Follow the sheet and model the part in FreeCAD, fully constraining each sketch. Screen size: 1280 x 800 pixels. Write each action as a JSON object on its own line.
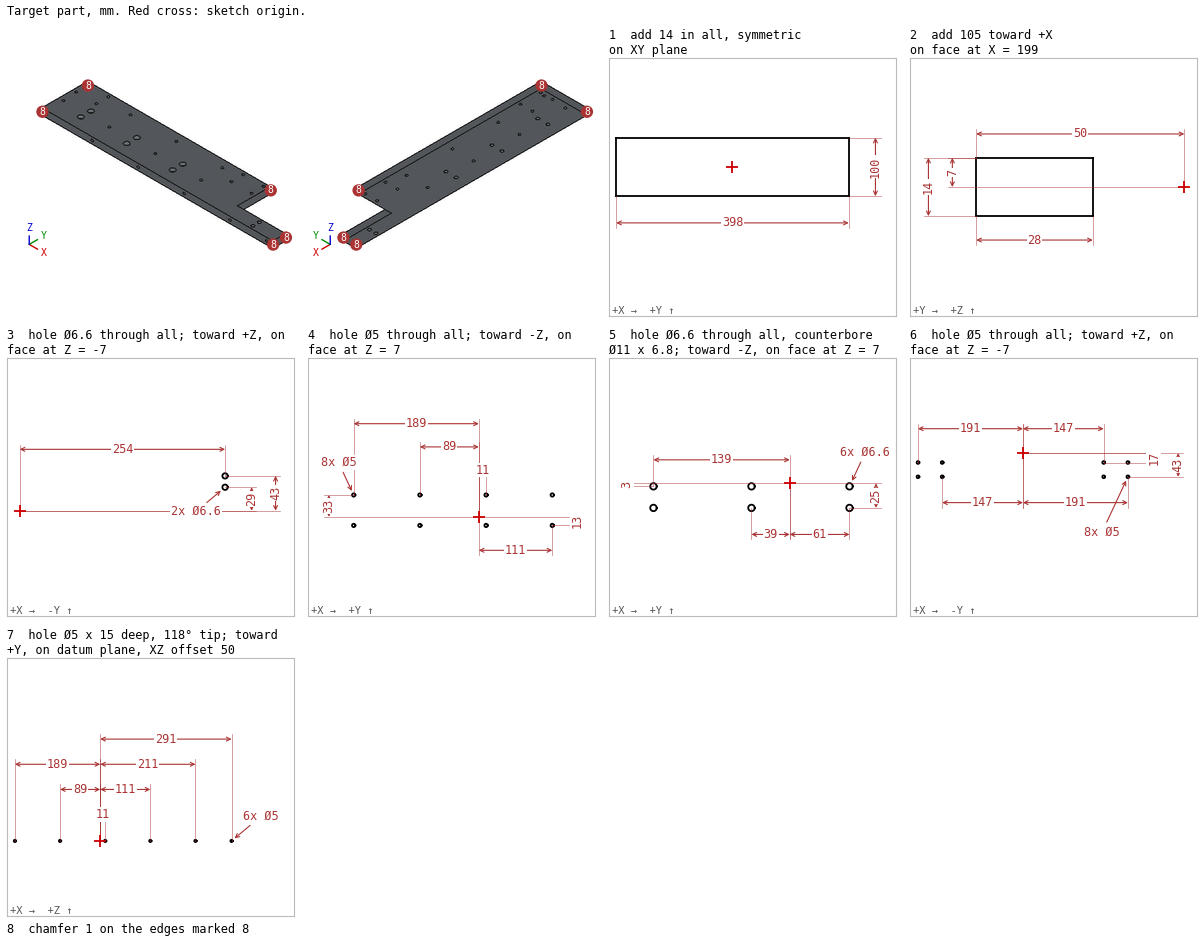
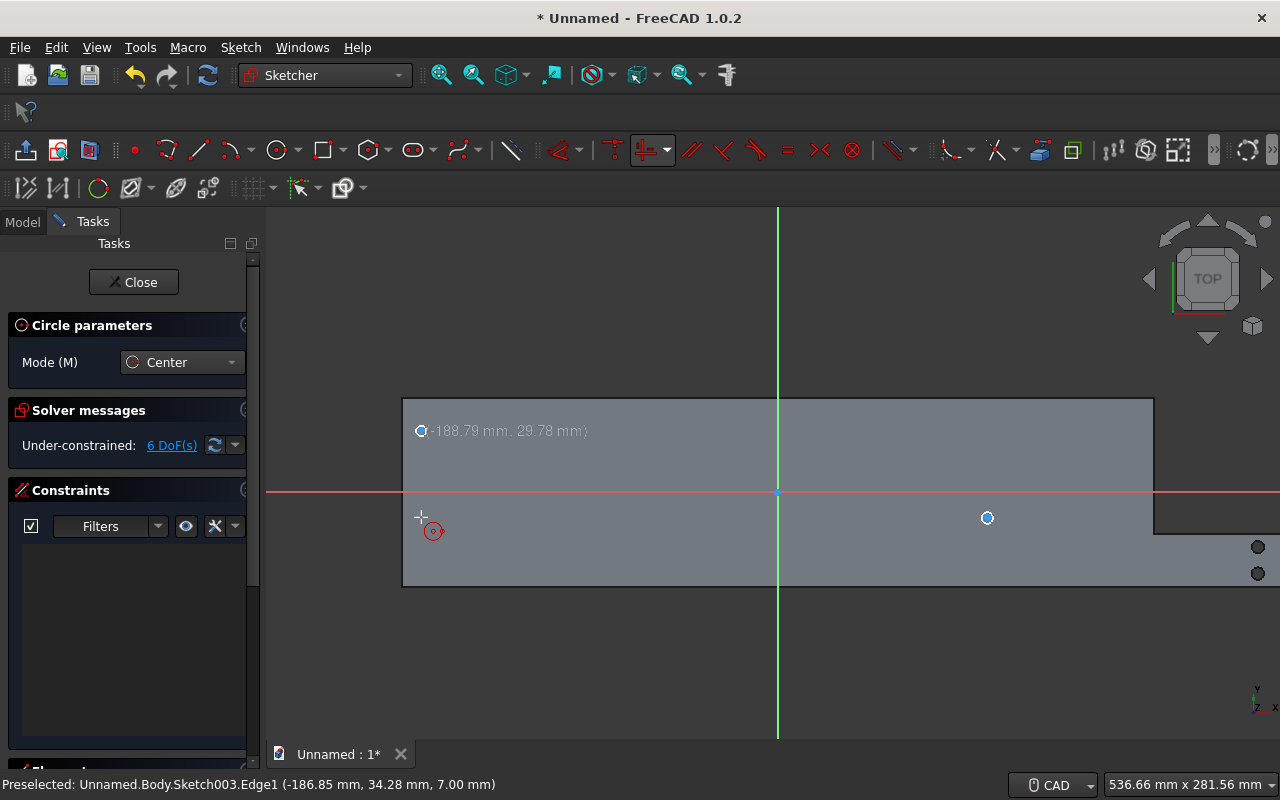
{"action": "left_click", "coordinate": [421, 517]}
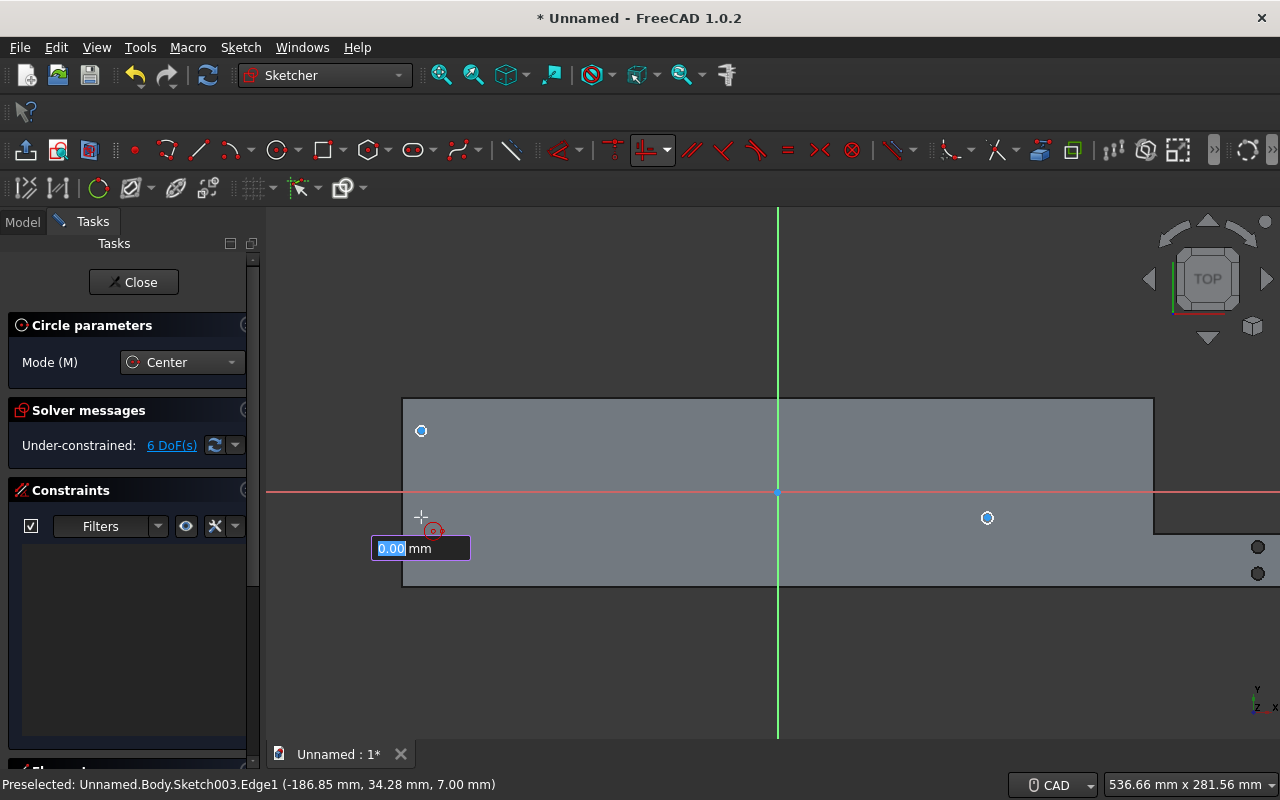
{"action": "scroll", "coordinate": [424, 514], "scroll_direction": "up", "scroll_amount": 7}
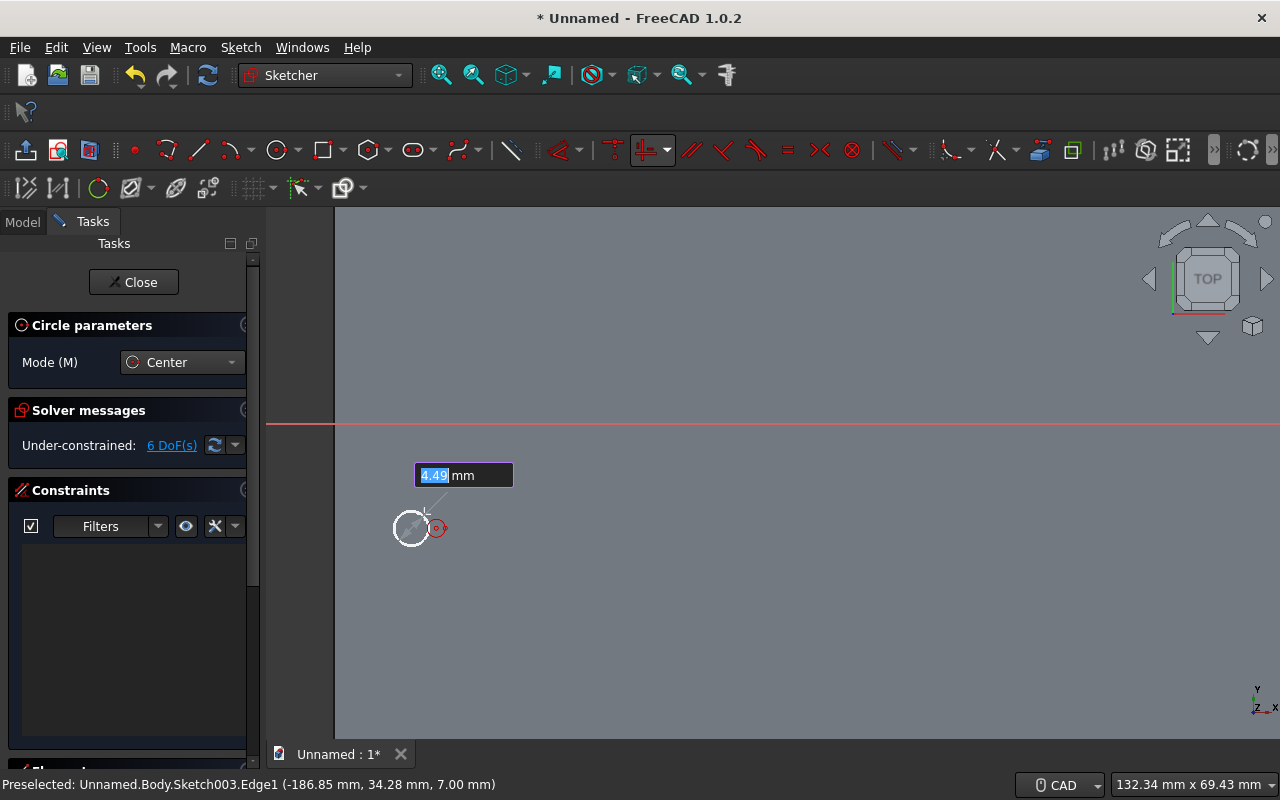
{"action": "left_click", "coordinate": [424, 510]}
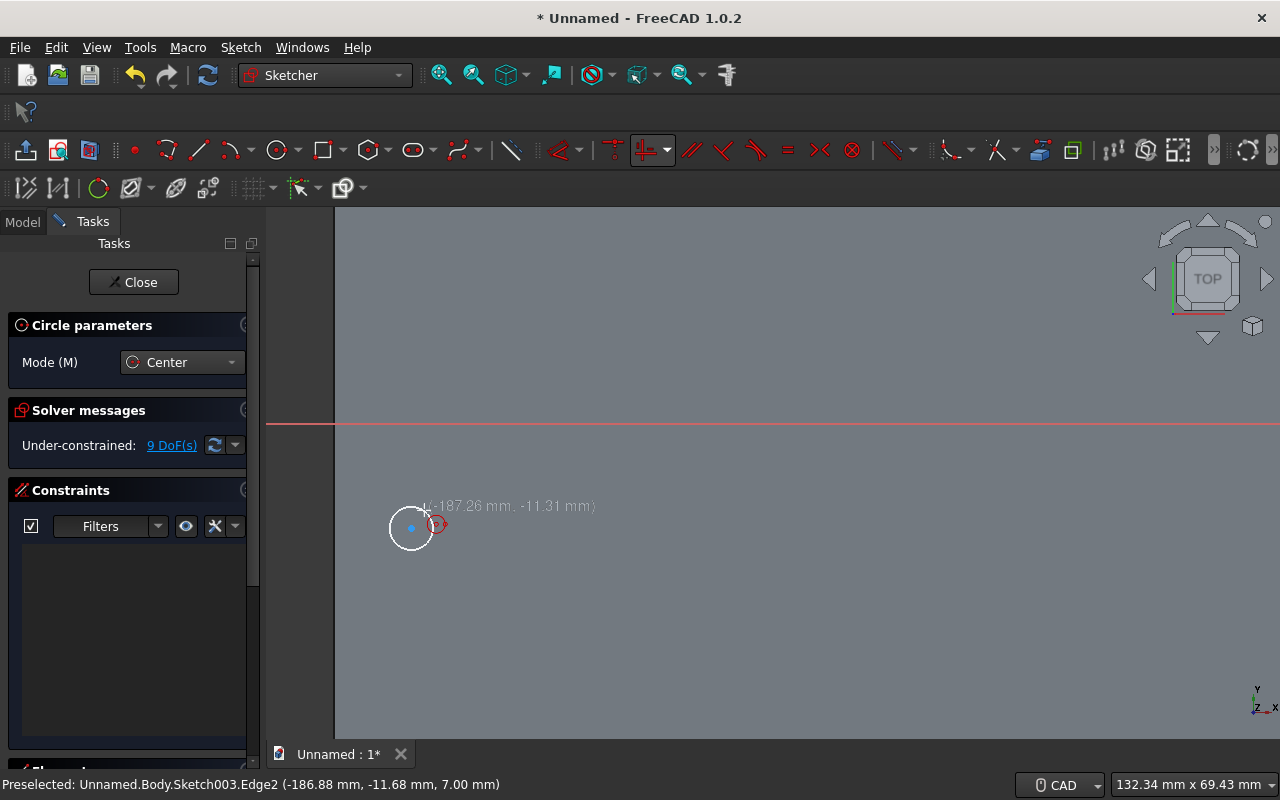
{"action": "scroll", "coordinate": [424, 514], "scroll_direction": "down", "scroll_amount": 7}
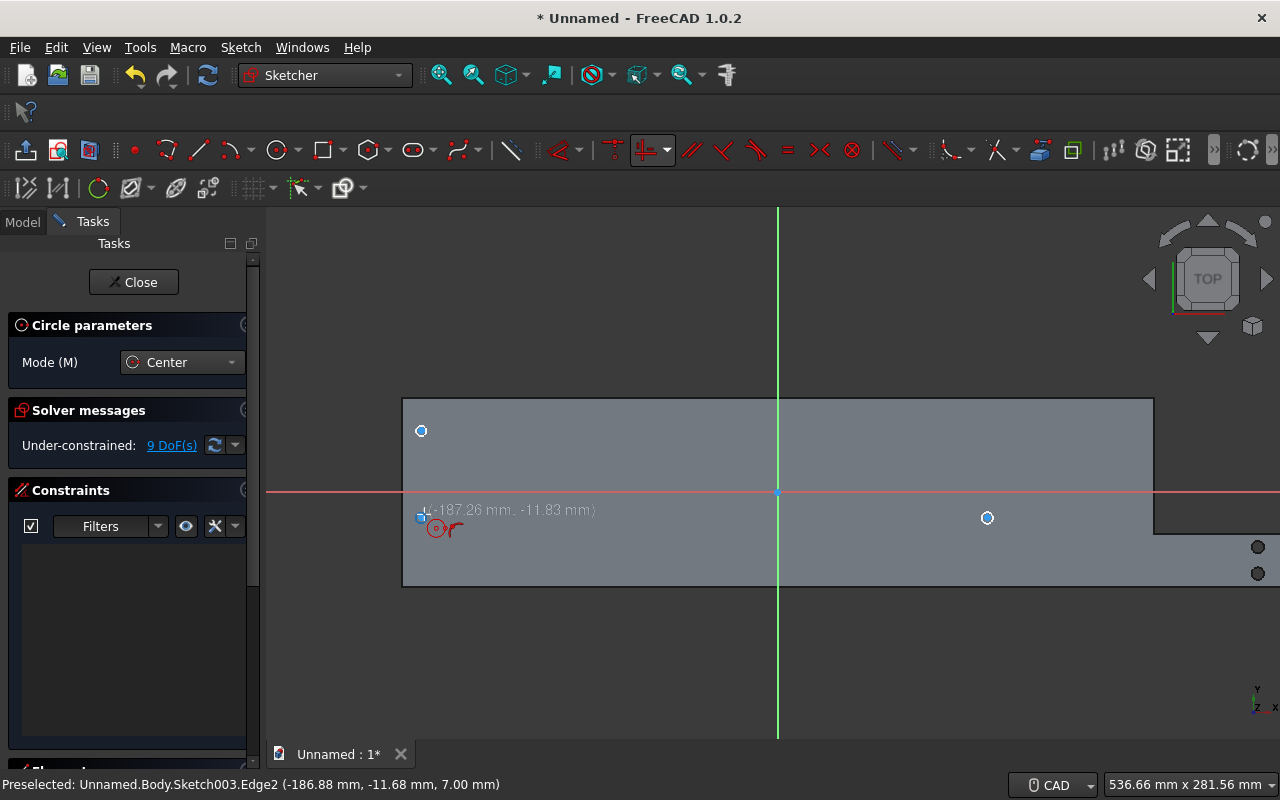
{"action": "scroll", "coordinate": [610, 430], "scroll_direction": "up", "scroll_amount": 8}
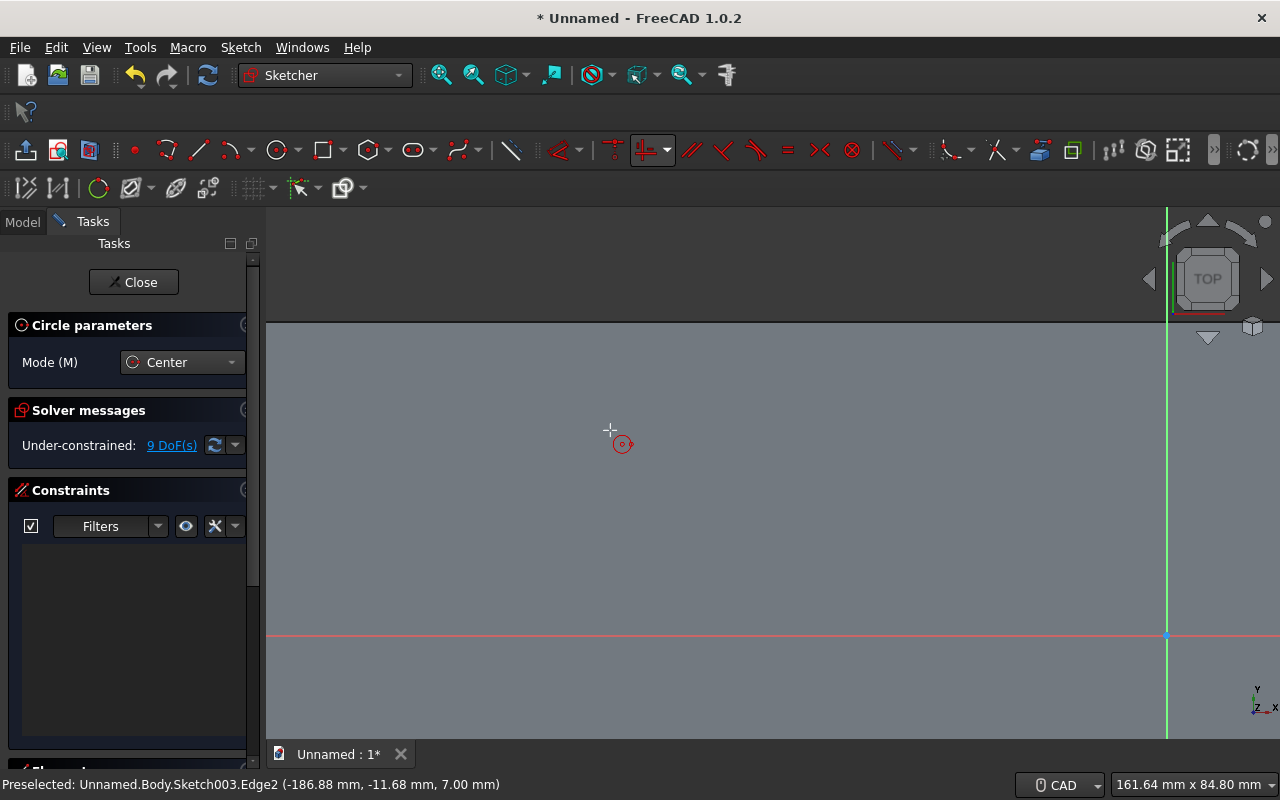
{"action": "scroll", "coordinate": [611, 430], "scroll_direction": "down", "scroll_amount": 8}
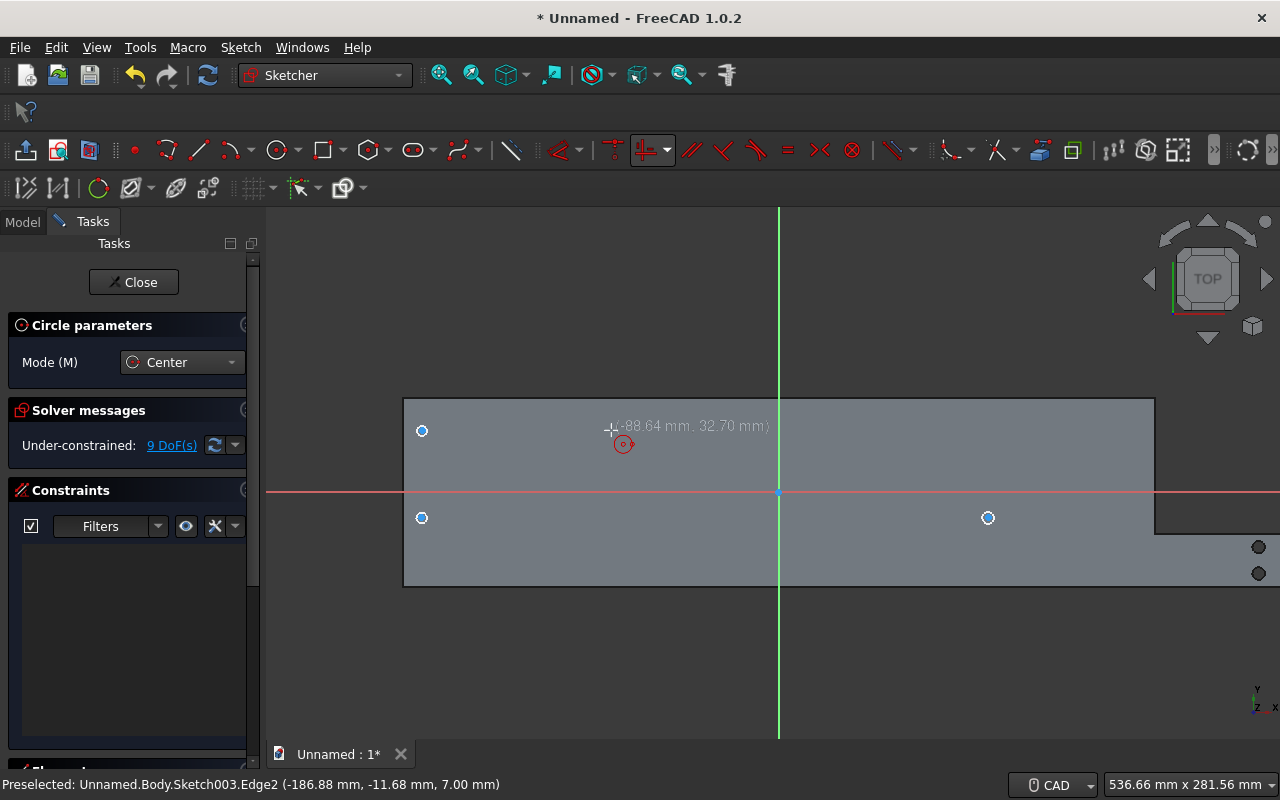
{"action": "left_click", "coordinate": [611, 430]}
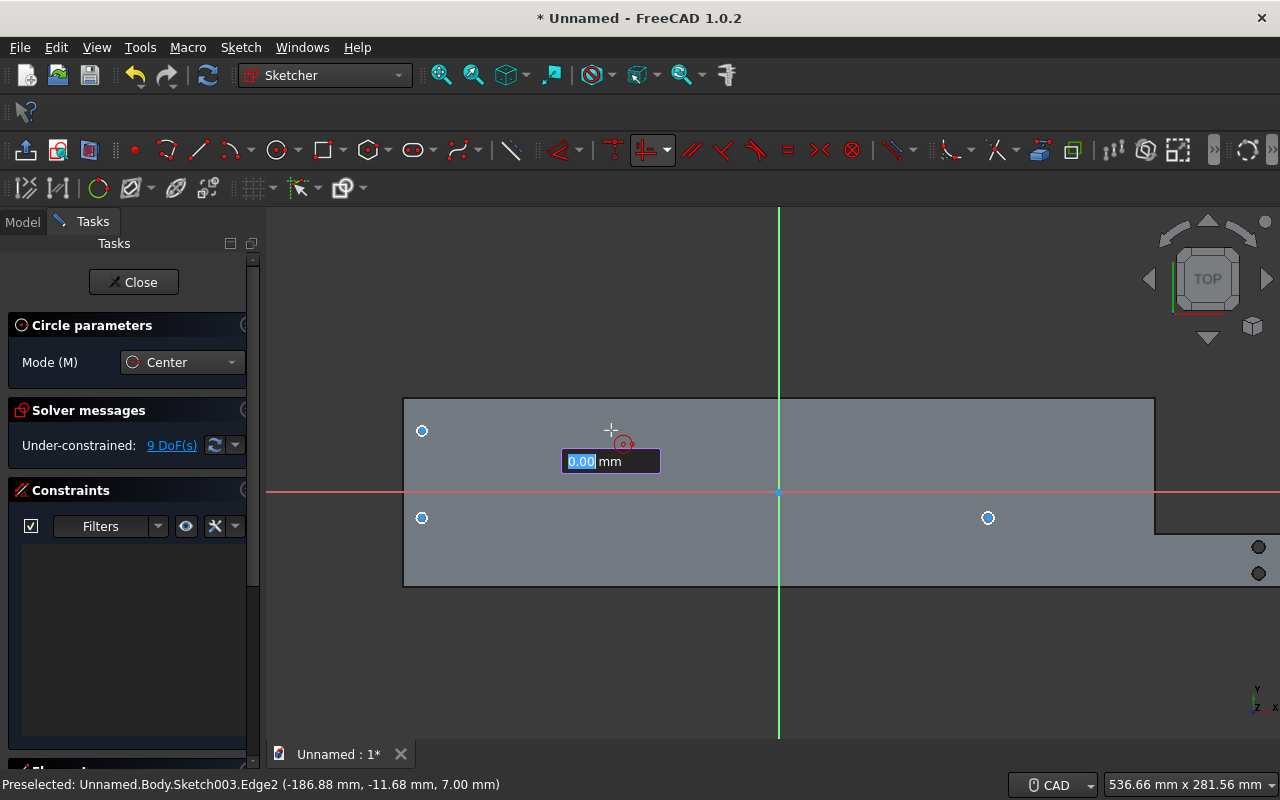
{"action": "scroll", "coordinate": [614, 427], "scroll_direction": "up", "scroll_amount": 7}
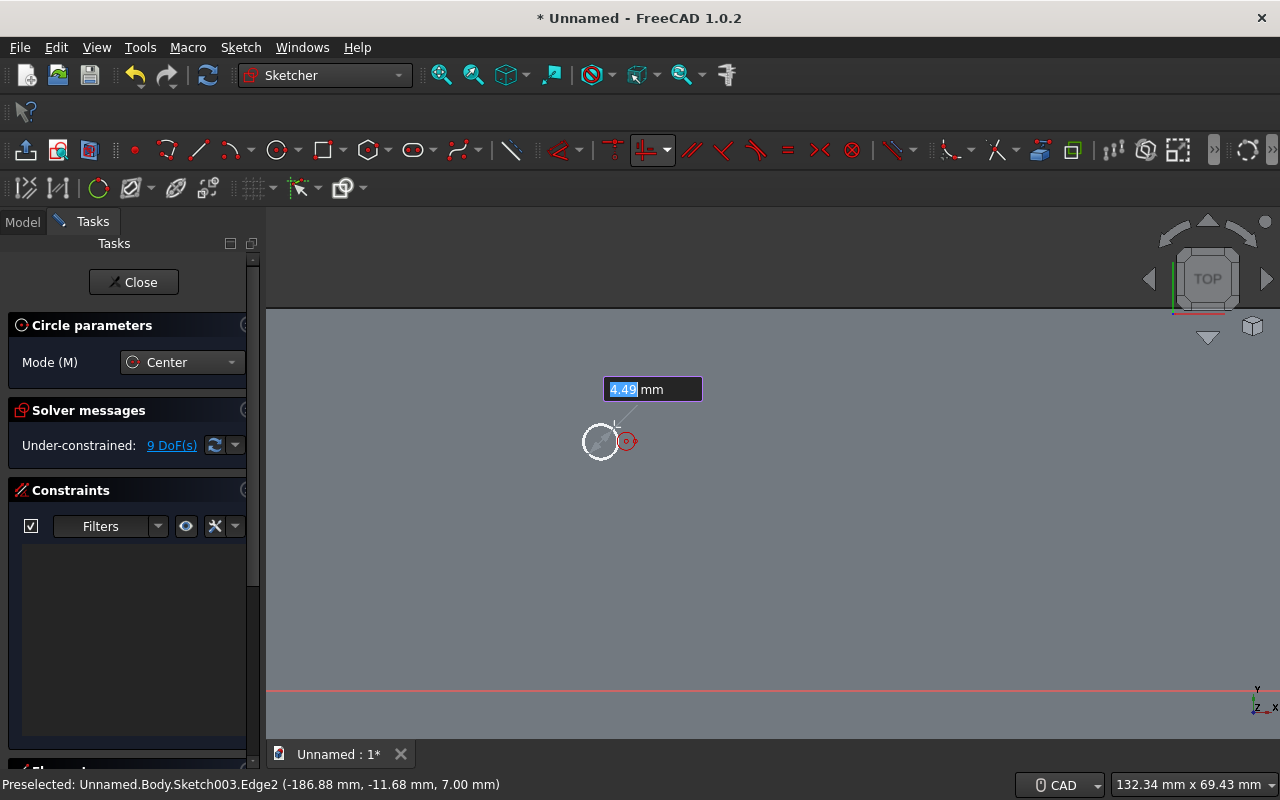
{"action": "left_click", "coordinate": [613, 424]}